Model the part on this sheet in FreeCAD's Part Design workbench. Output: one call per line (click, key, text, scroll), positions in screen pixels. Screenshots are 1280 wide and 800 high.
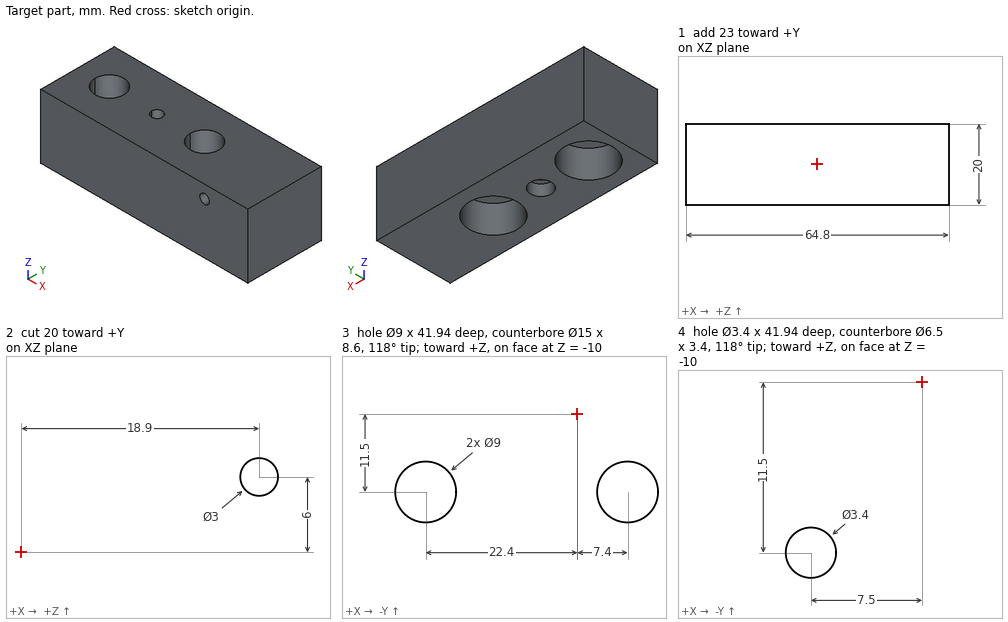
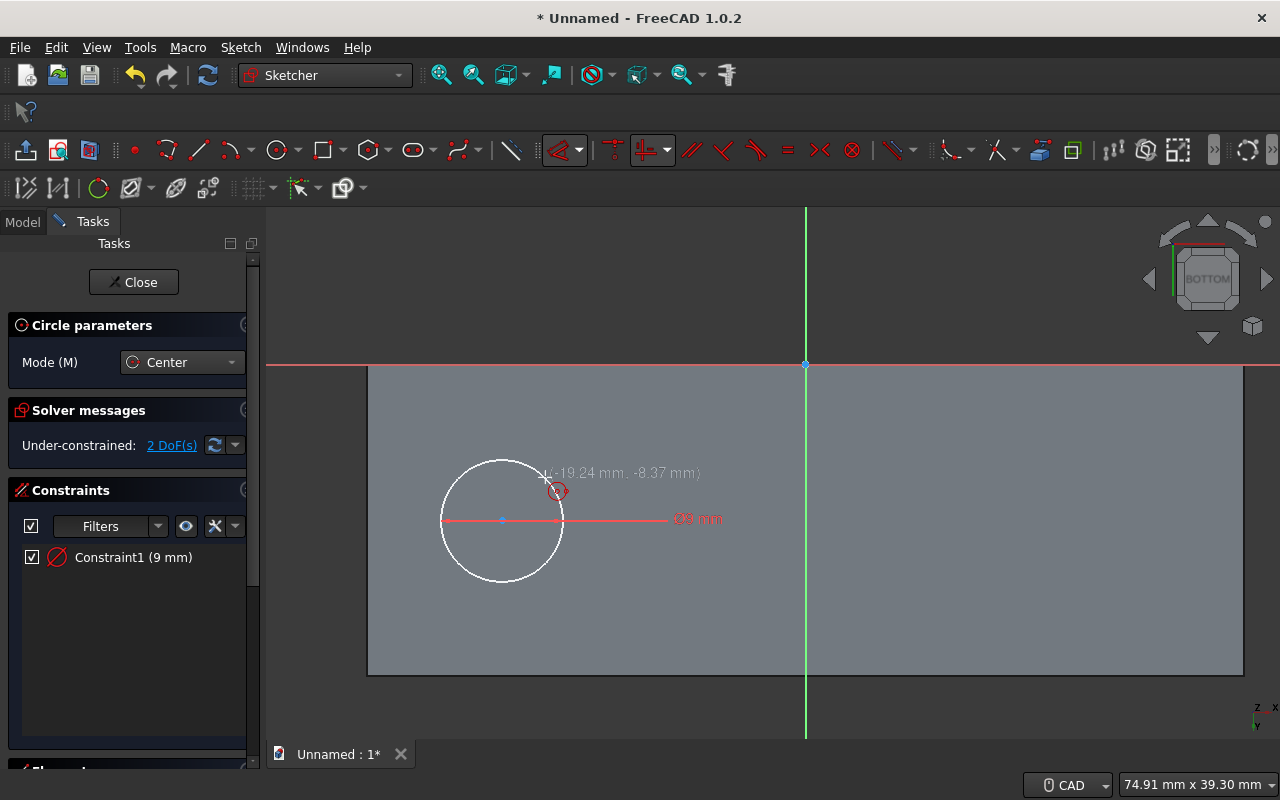
click(906, 520)
move(949, 477)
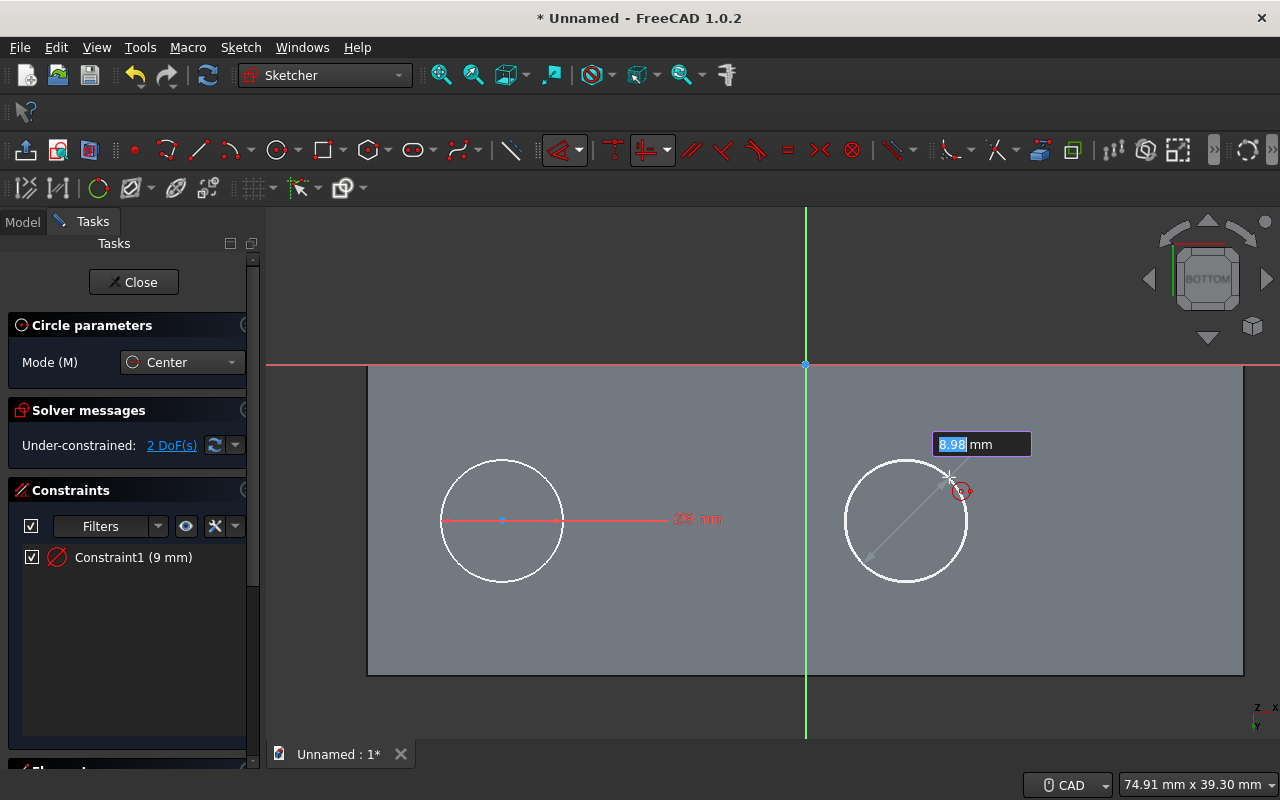
text(9)
key(Return)
key(Escape)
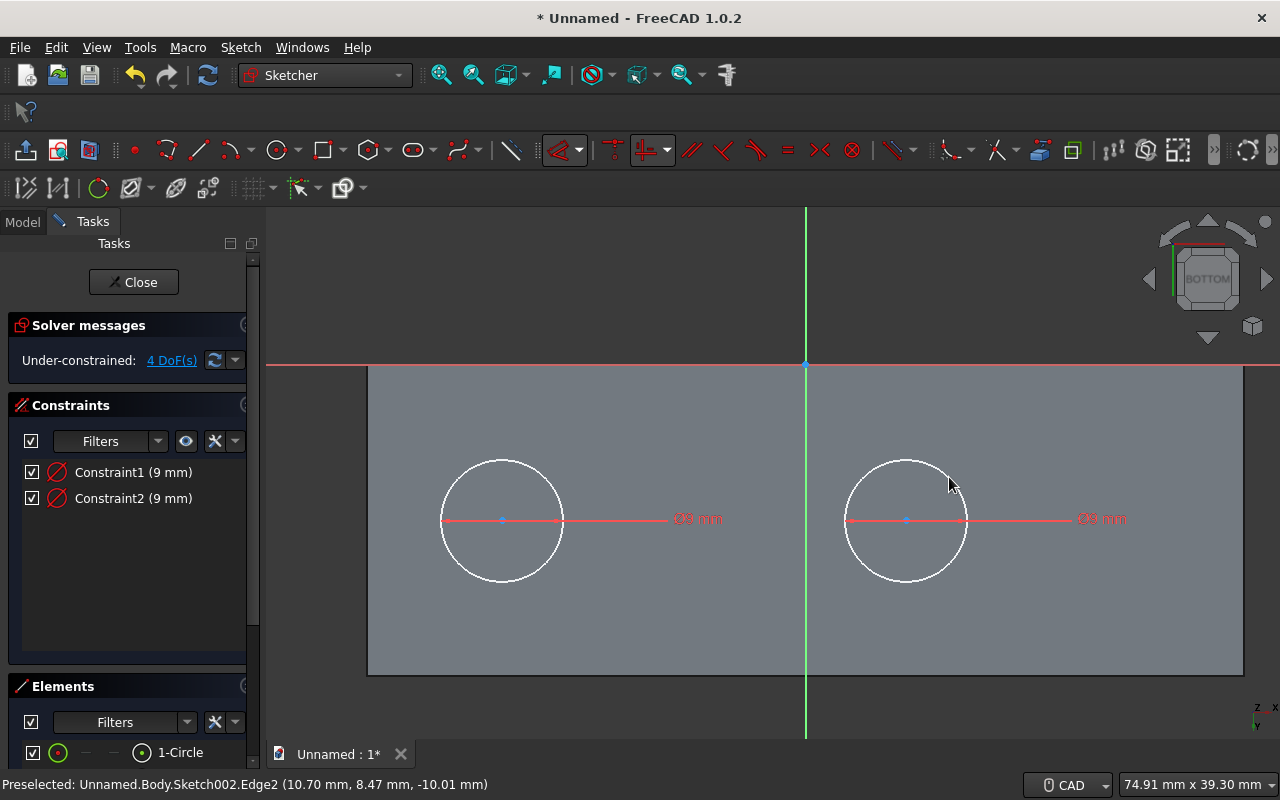
click(502, 521)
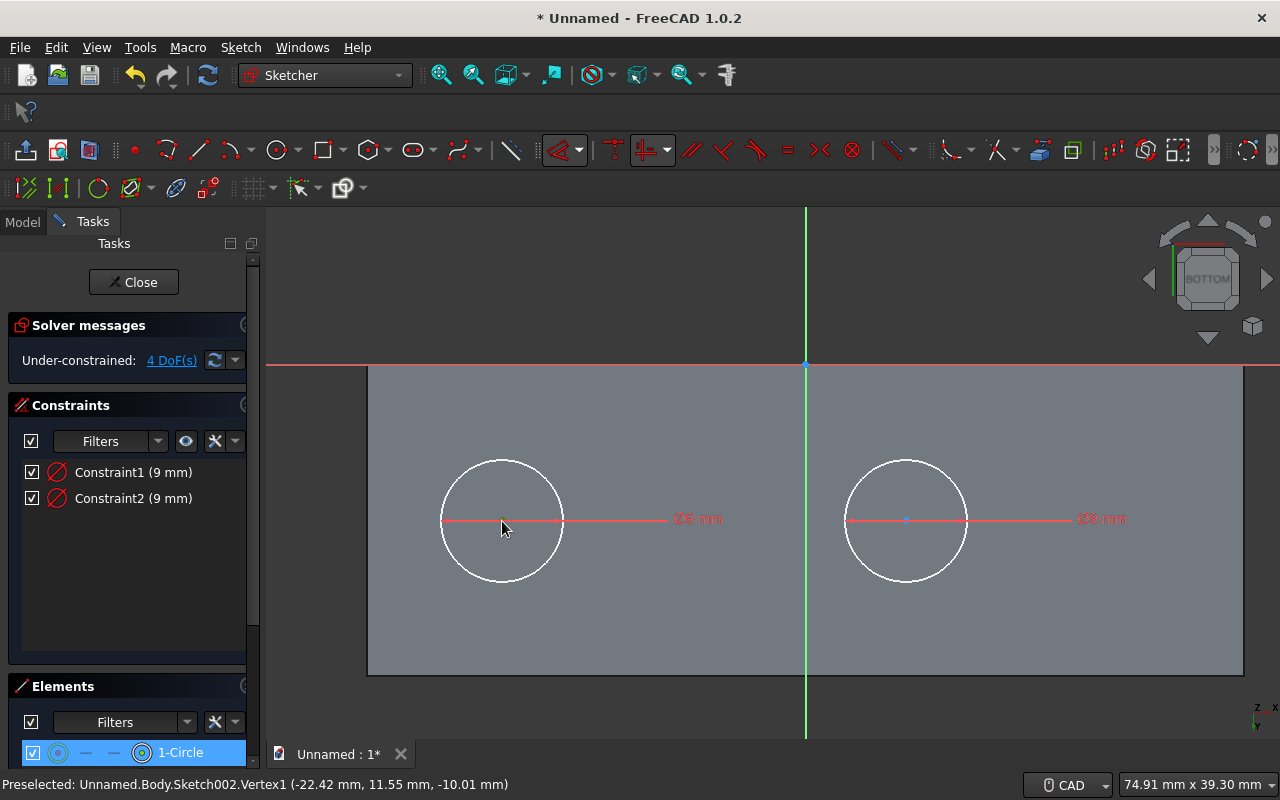
click(906, 521)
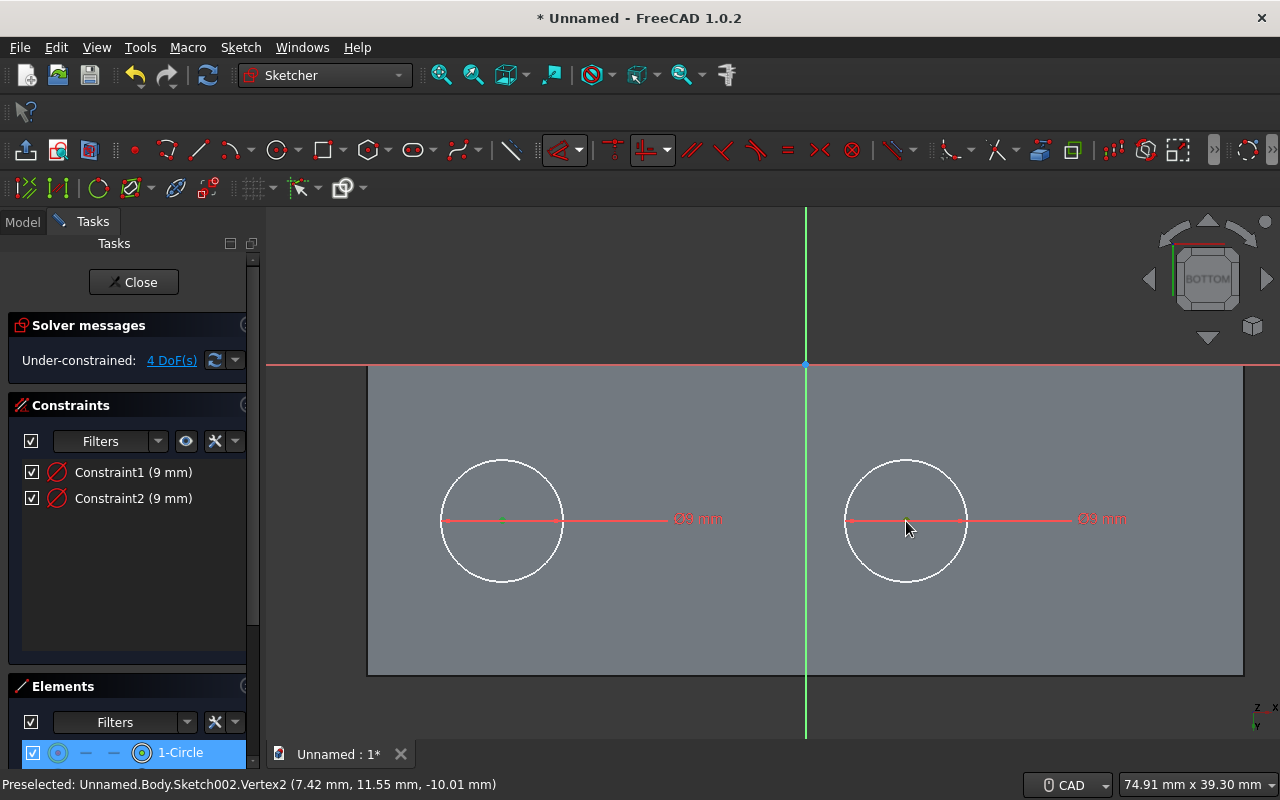
key(h)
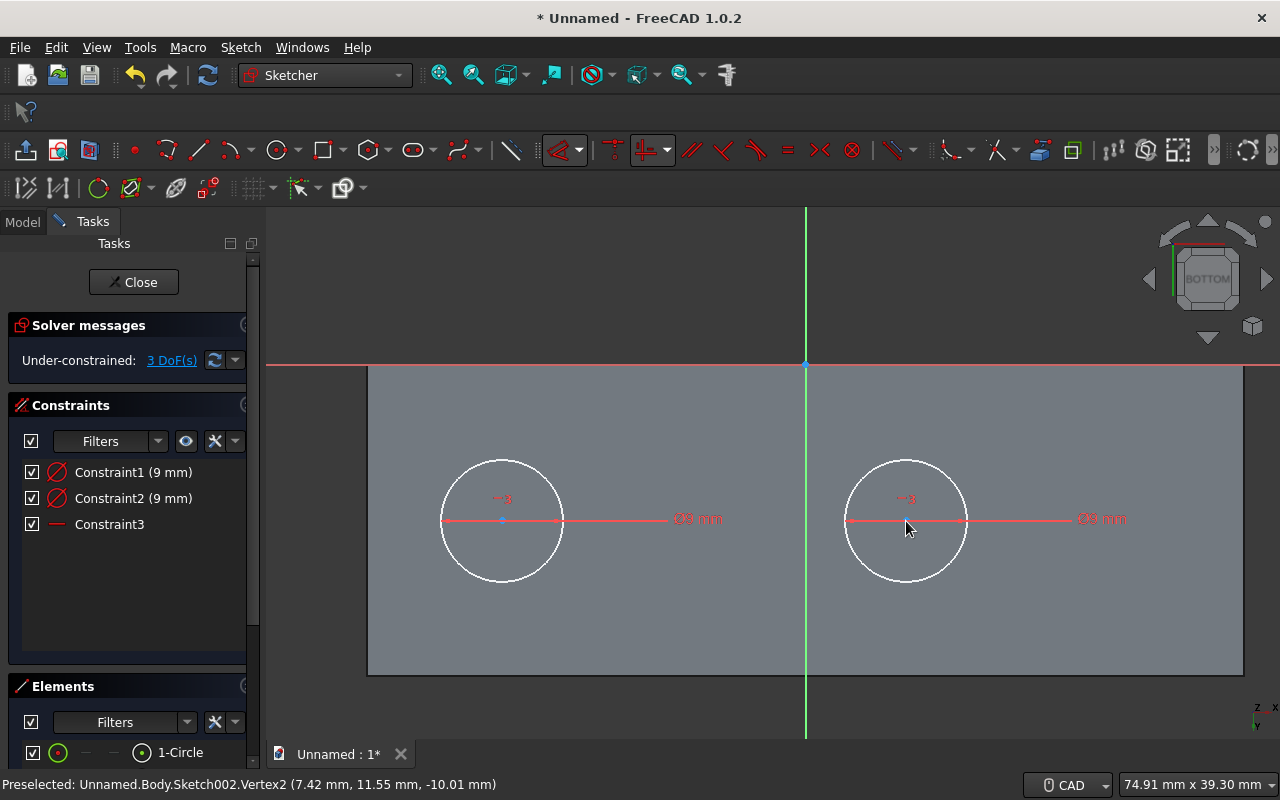
click(906, 521)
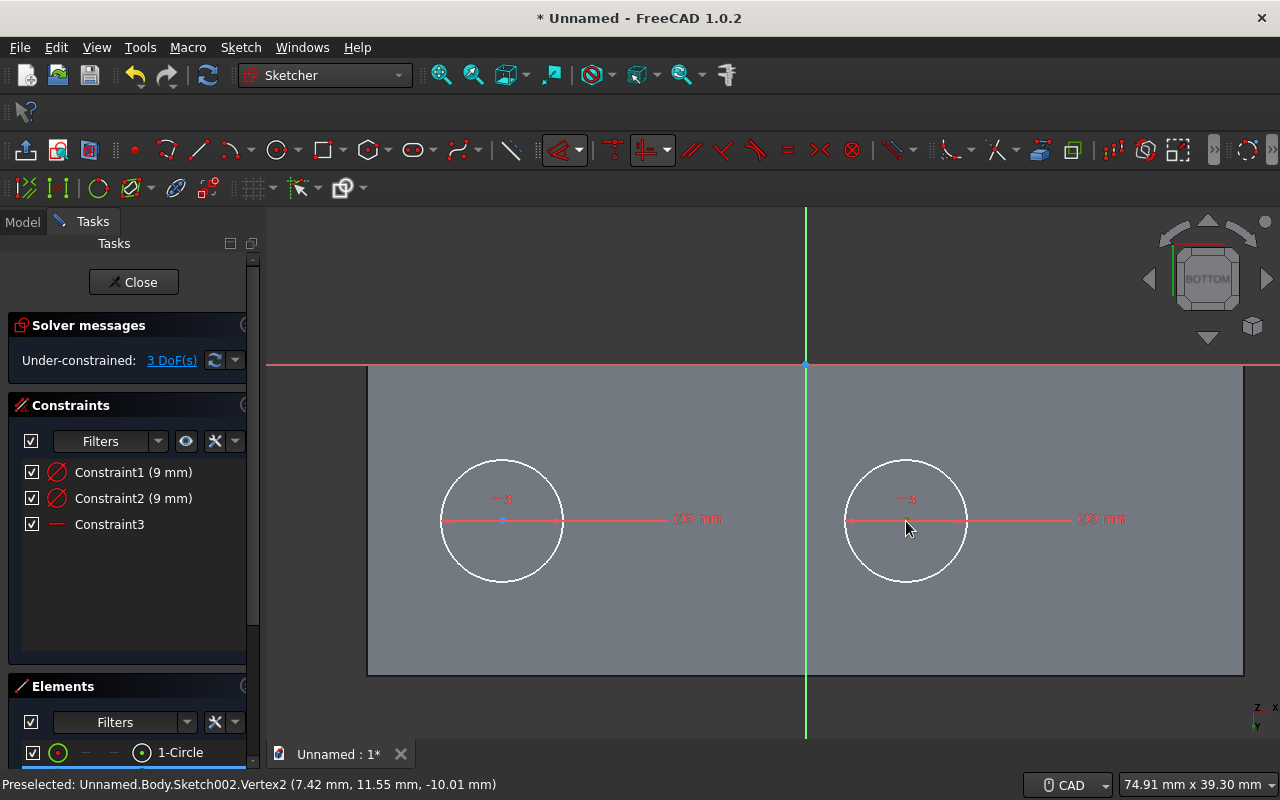
click(582, 150)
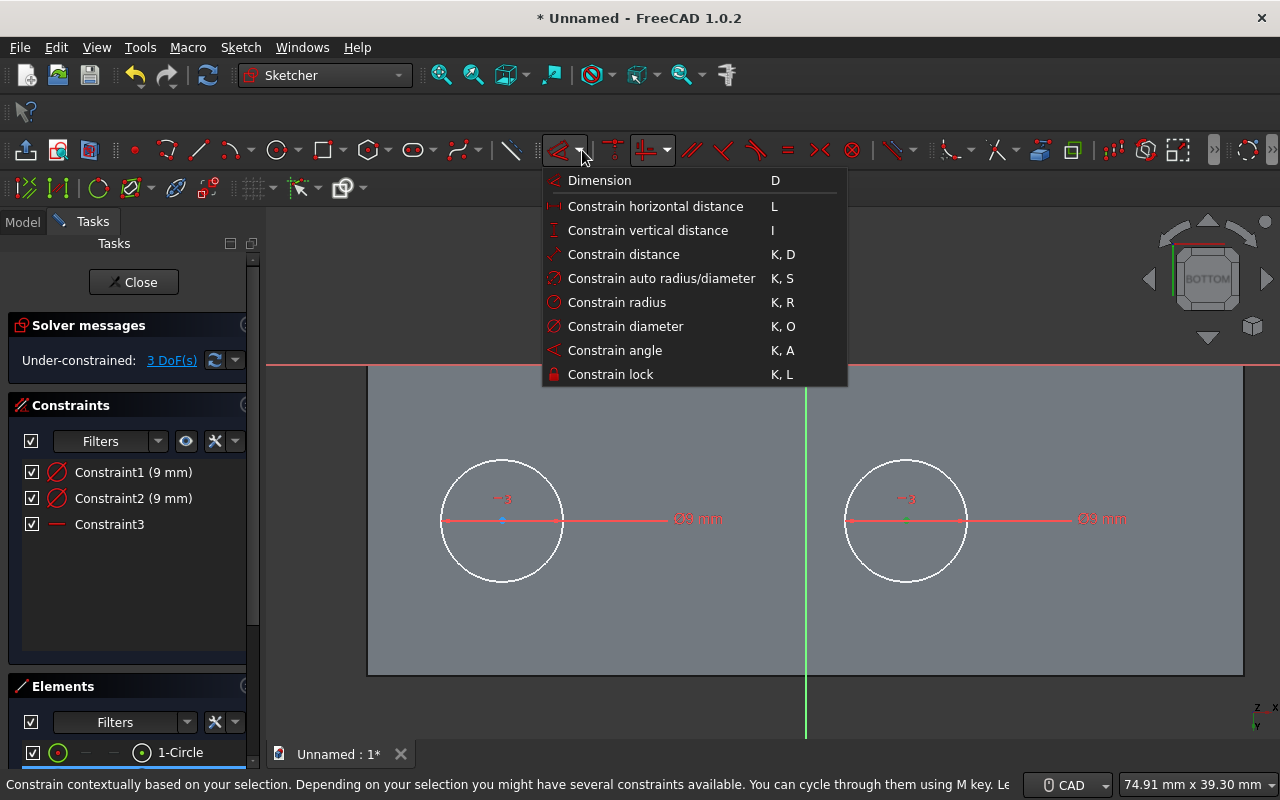
click(695, 206)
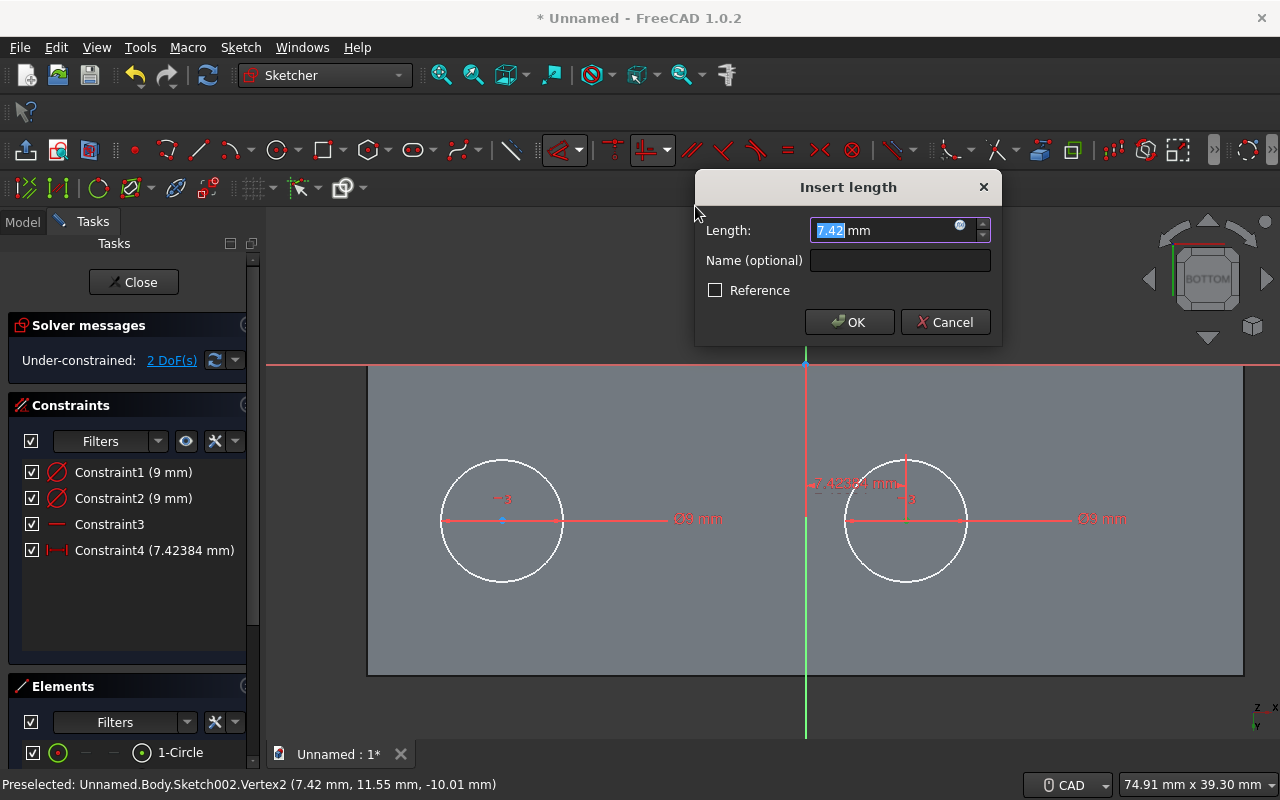
text(7.4)
key(Return)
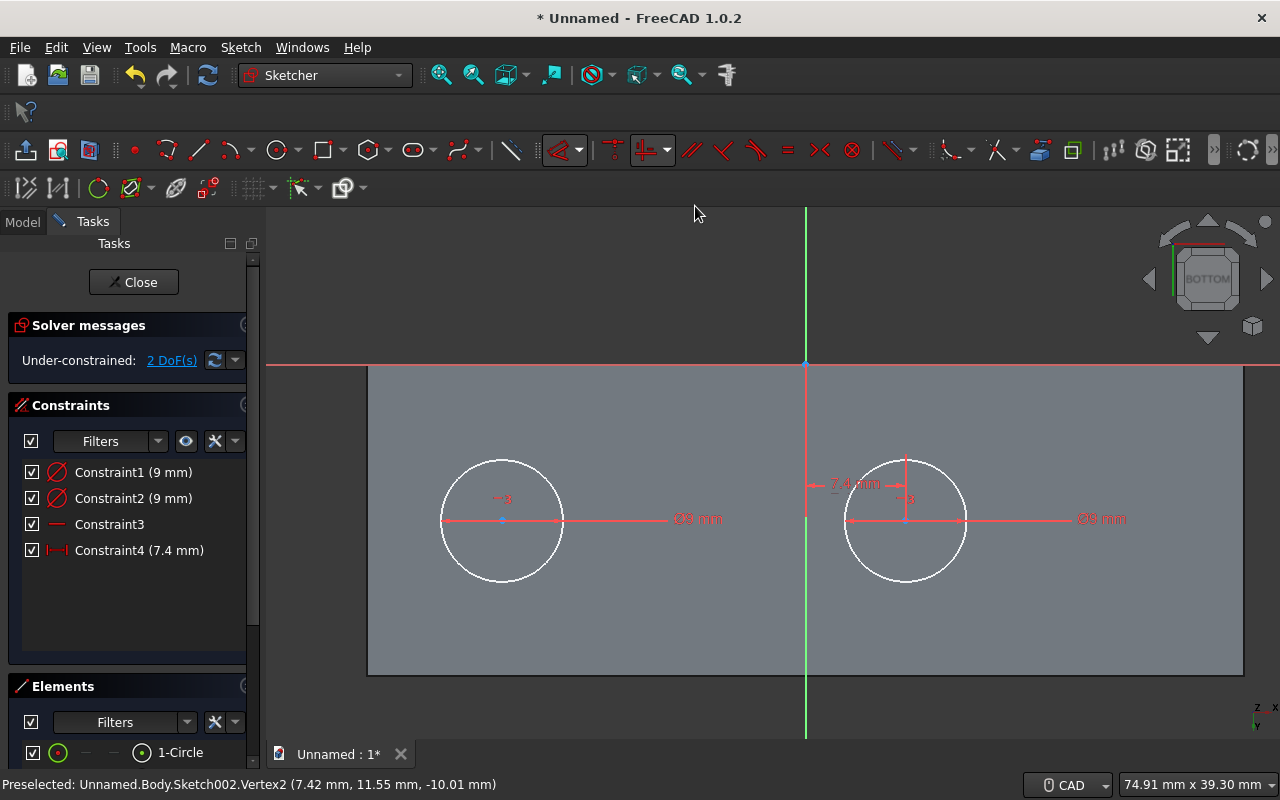
click(502, 521)